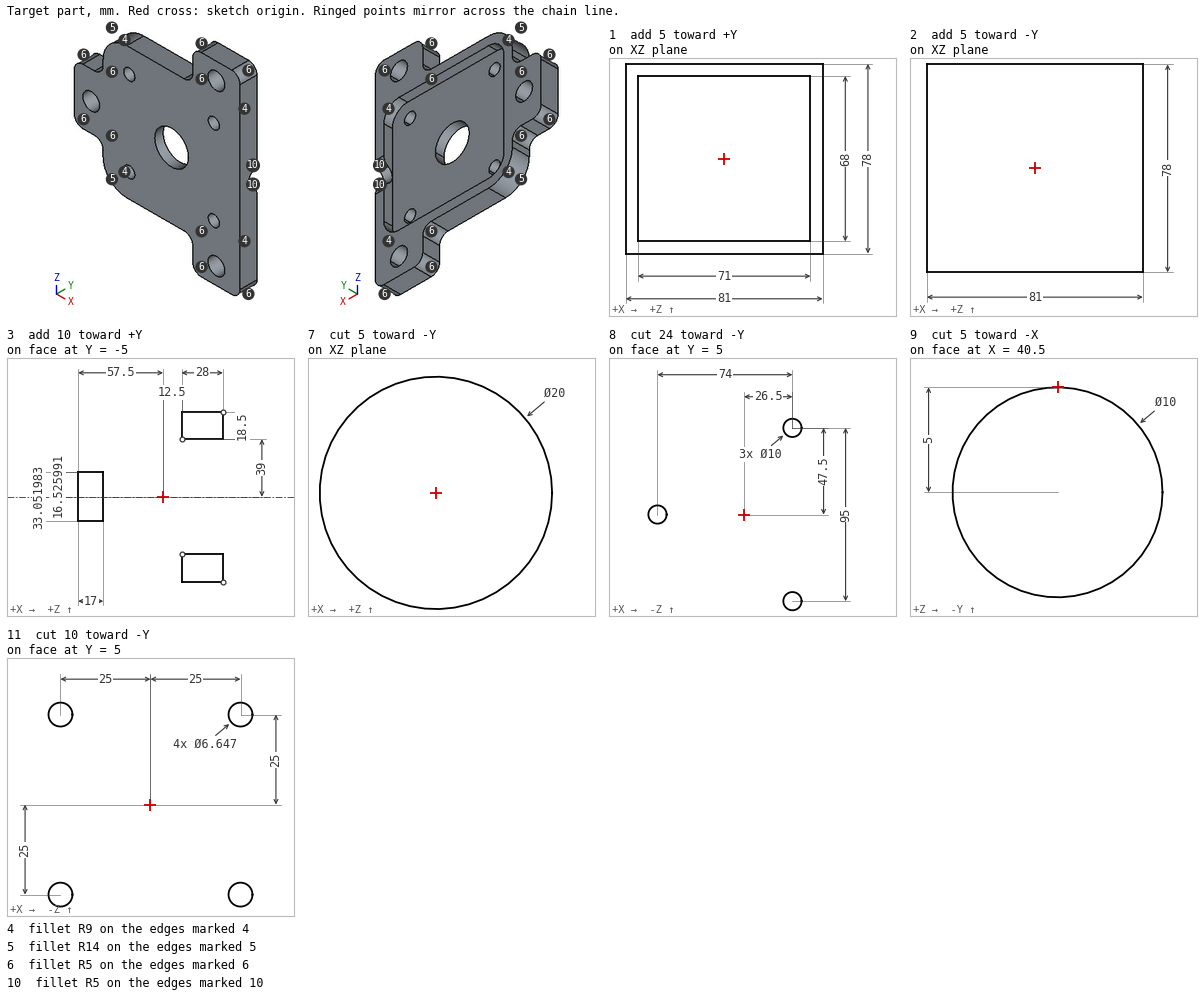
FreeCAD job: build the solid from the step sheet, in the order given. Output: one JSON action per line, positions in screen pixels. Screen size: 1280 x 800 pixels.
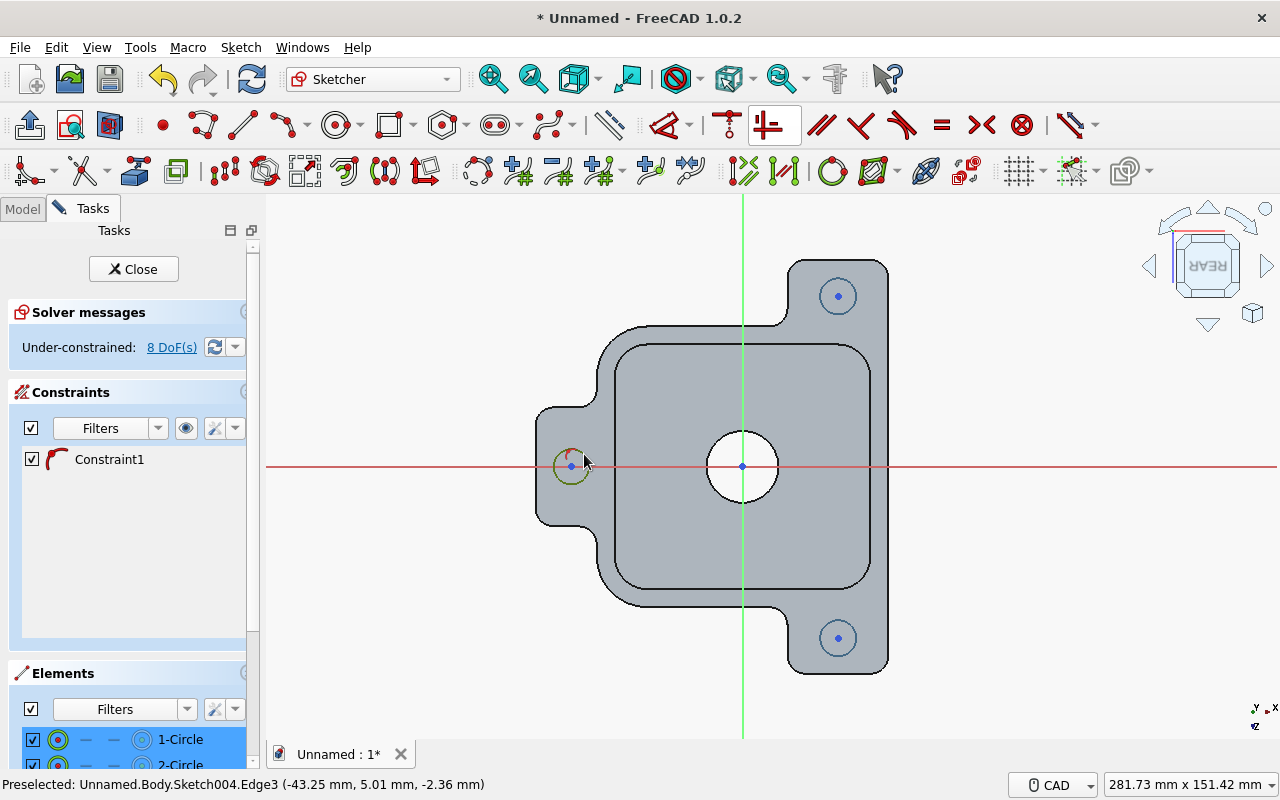
{"action": "left_click", "coordinate": [942, 126]}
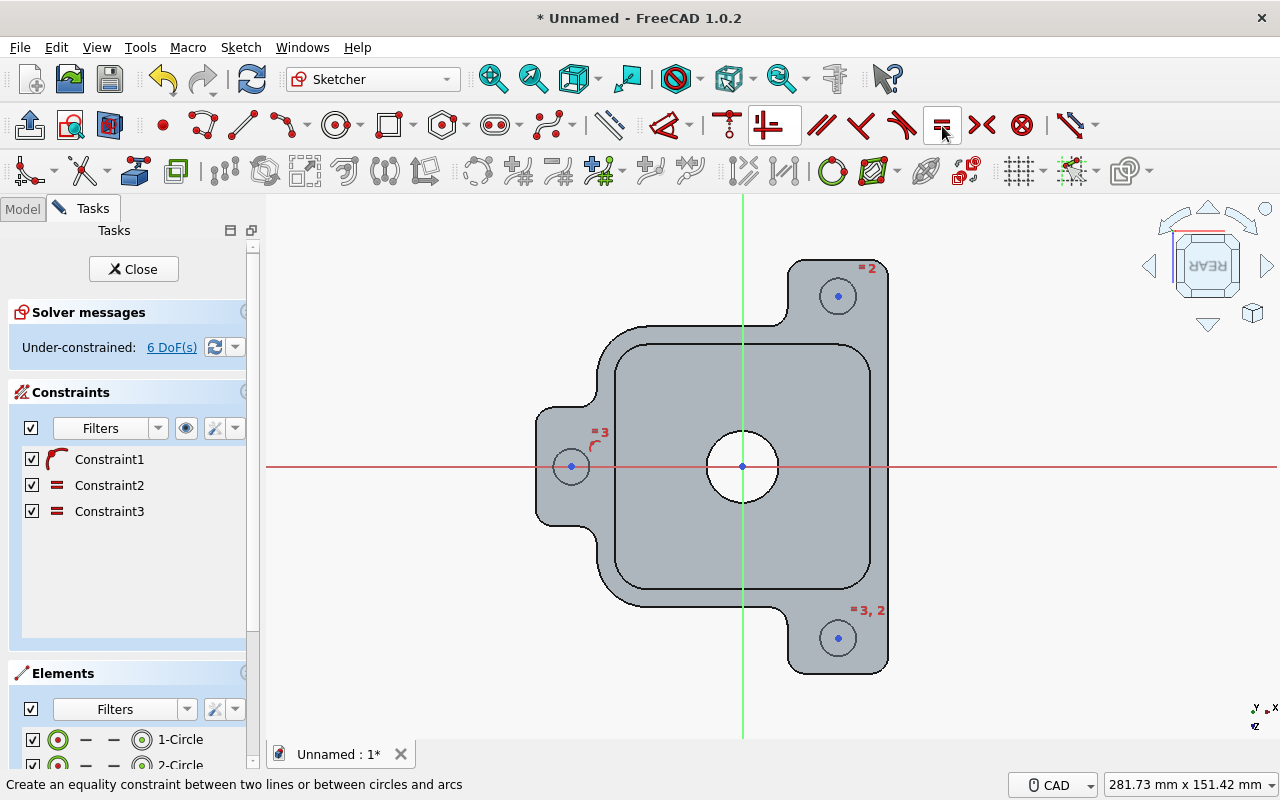
{"action": "left_click", "coordinate": [838, 296]}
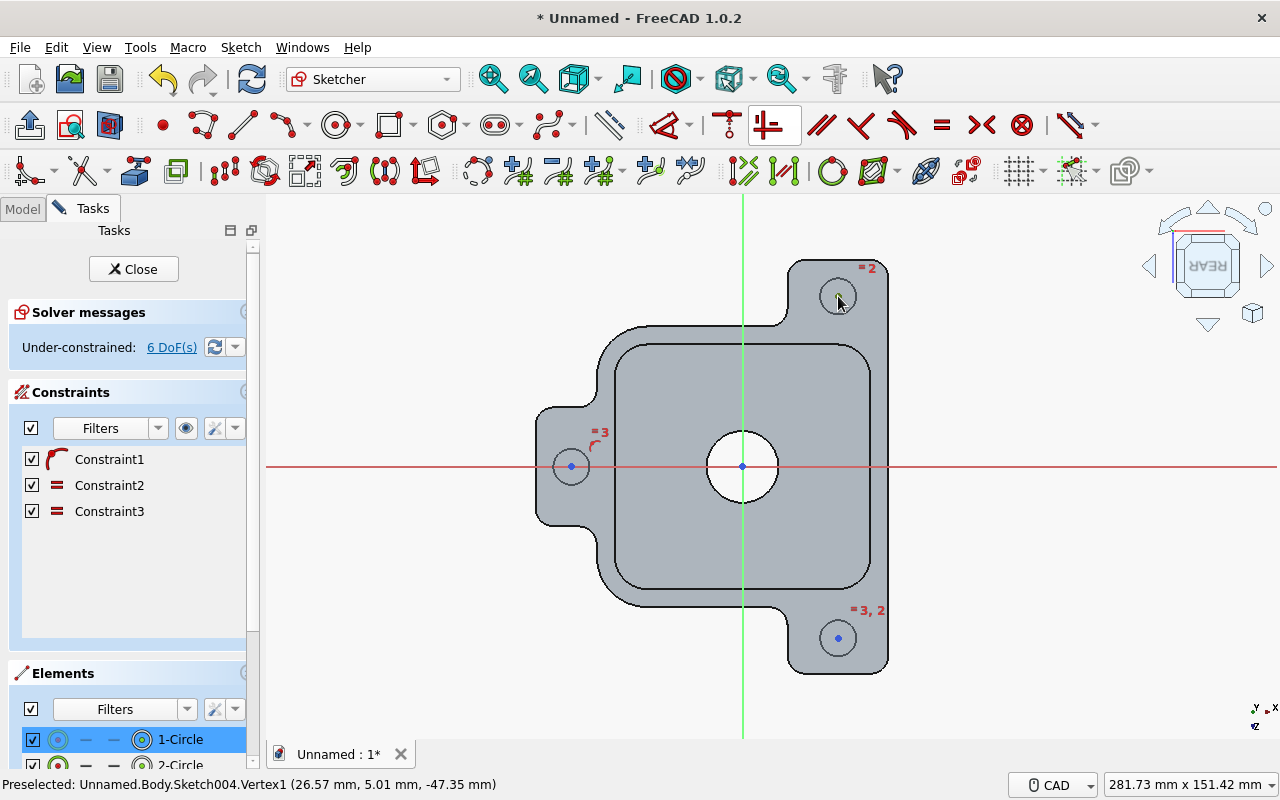
{"action": "left_click", "coordinate": [838, 638]}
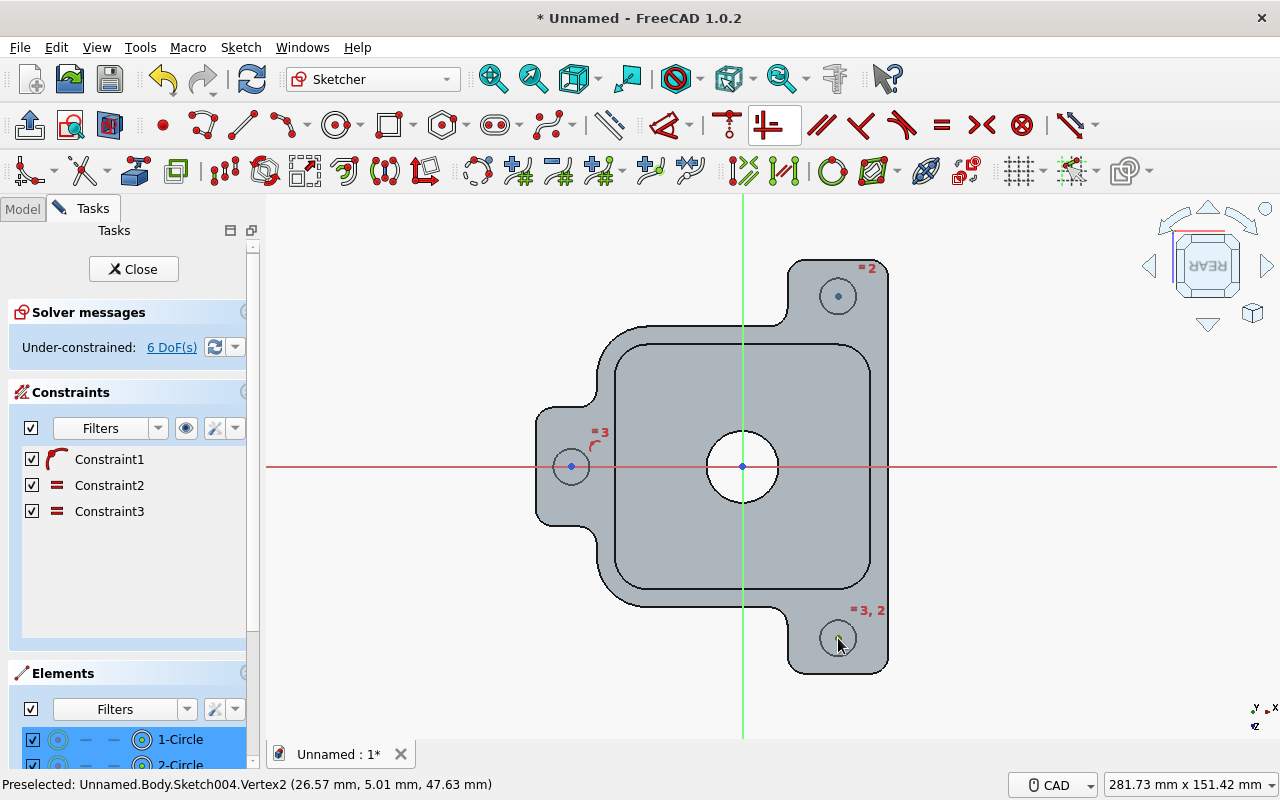
{"action": "key", "text": "v"}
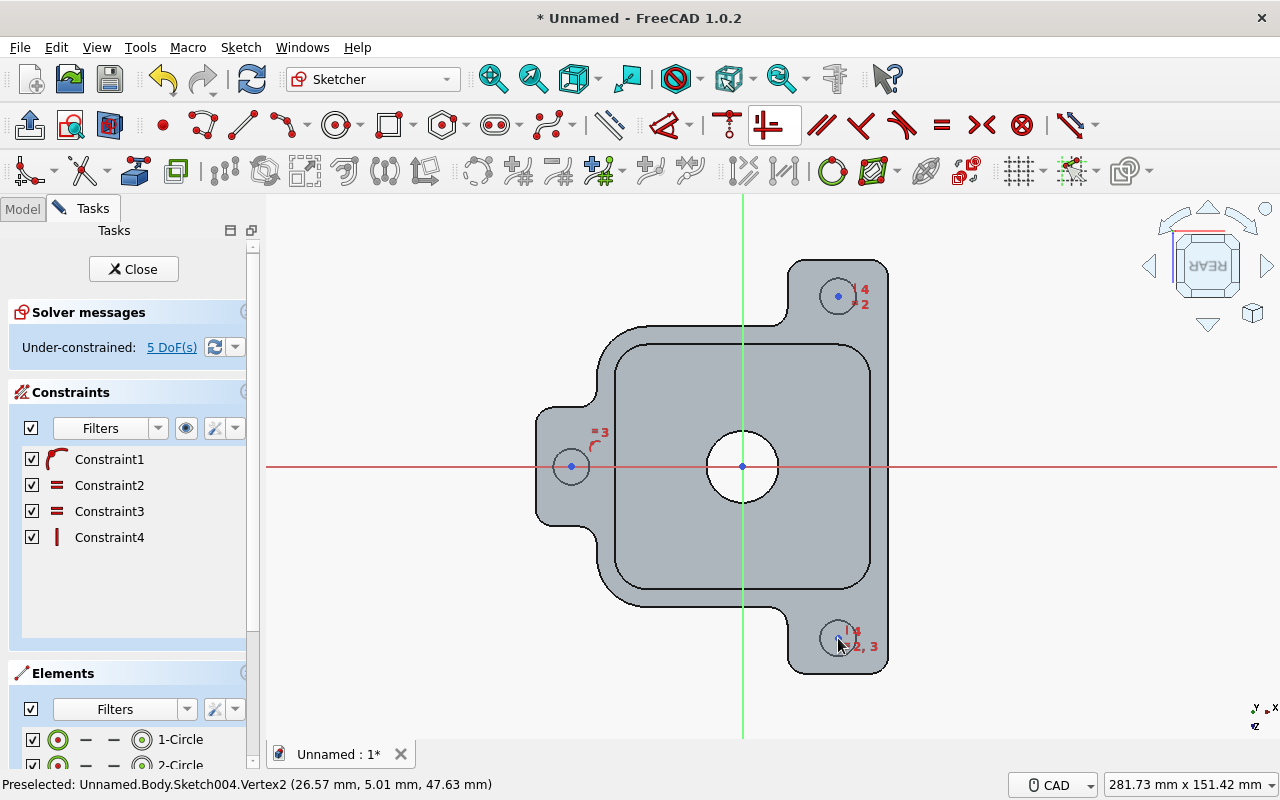
{"action": "left_click", "coordinate": [664, 126]}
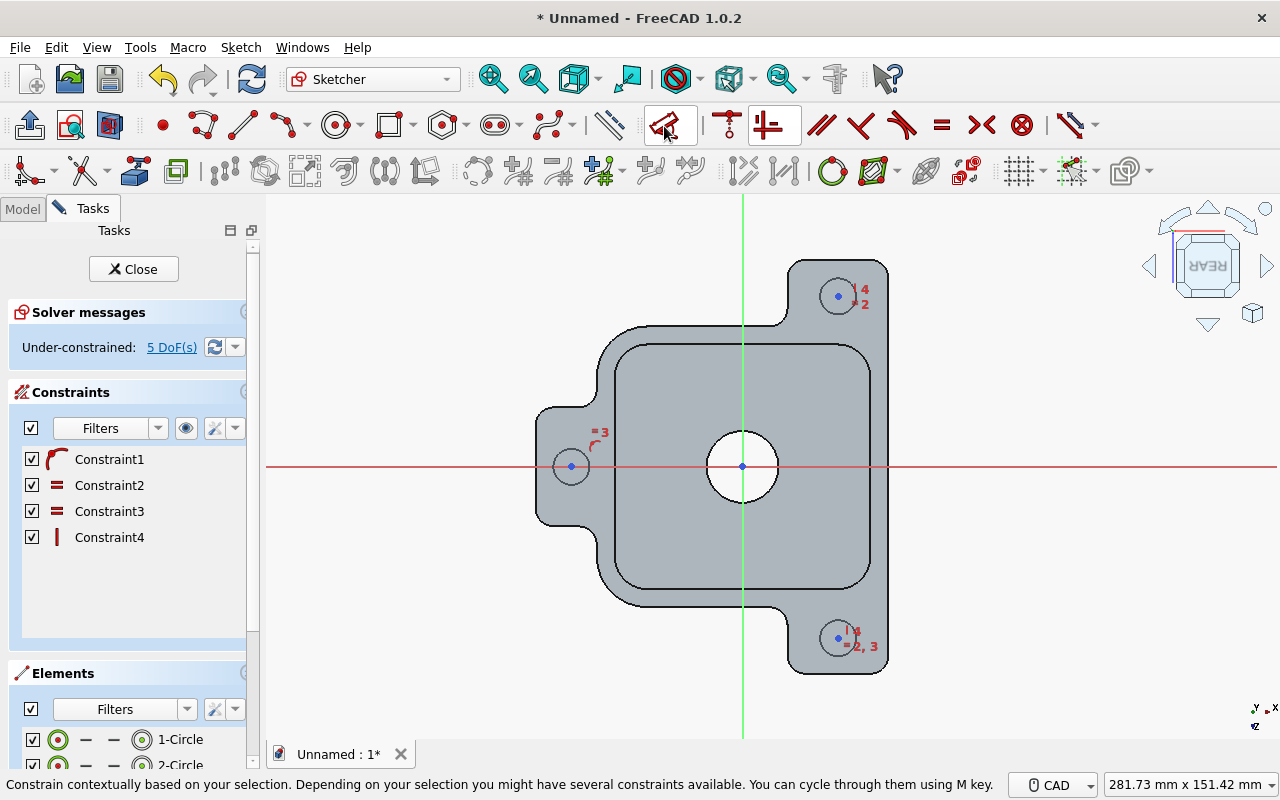
{"action": "left_click", "coordinate": [851, 284]}
{"action": "left_click", "coordinate": [874, 262]}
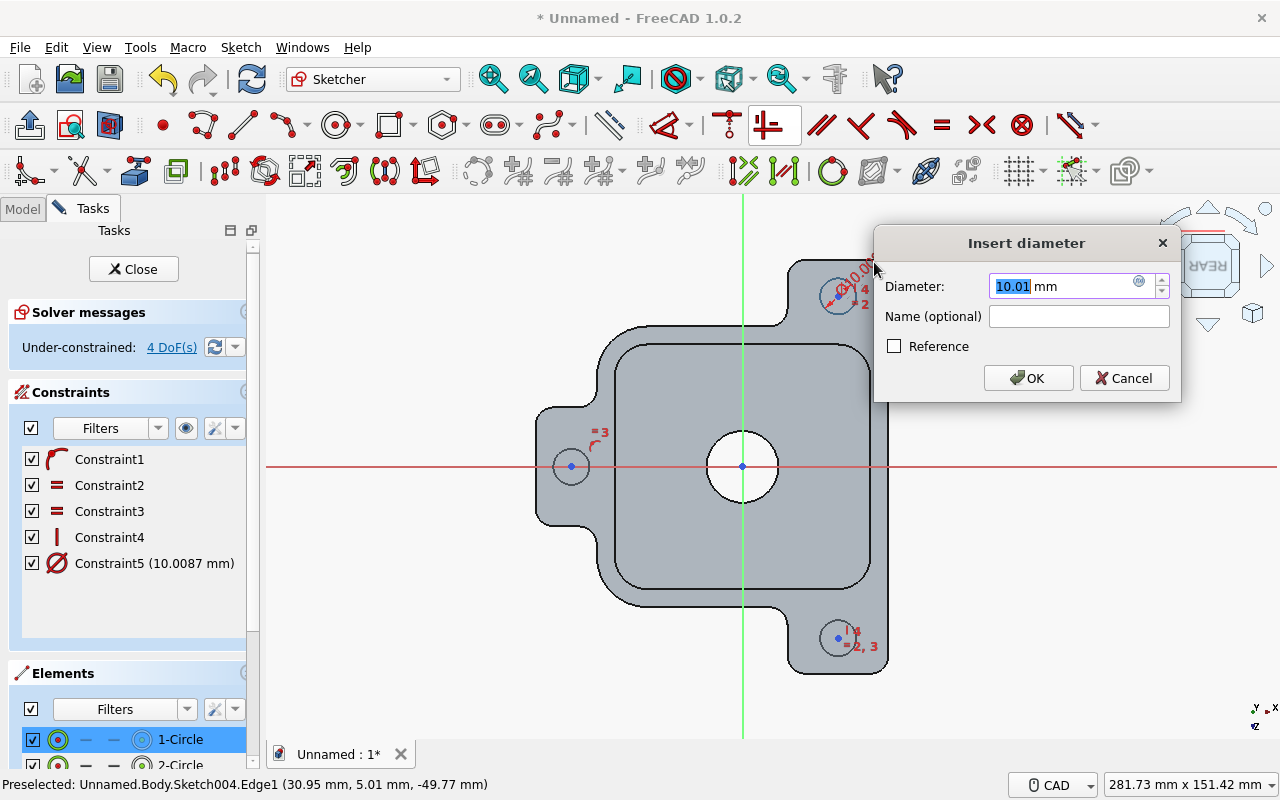
{"action": "type", "text": "10"}
{"action": "key", "text": "Return"}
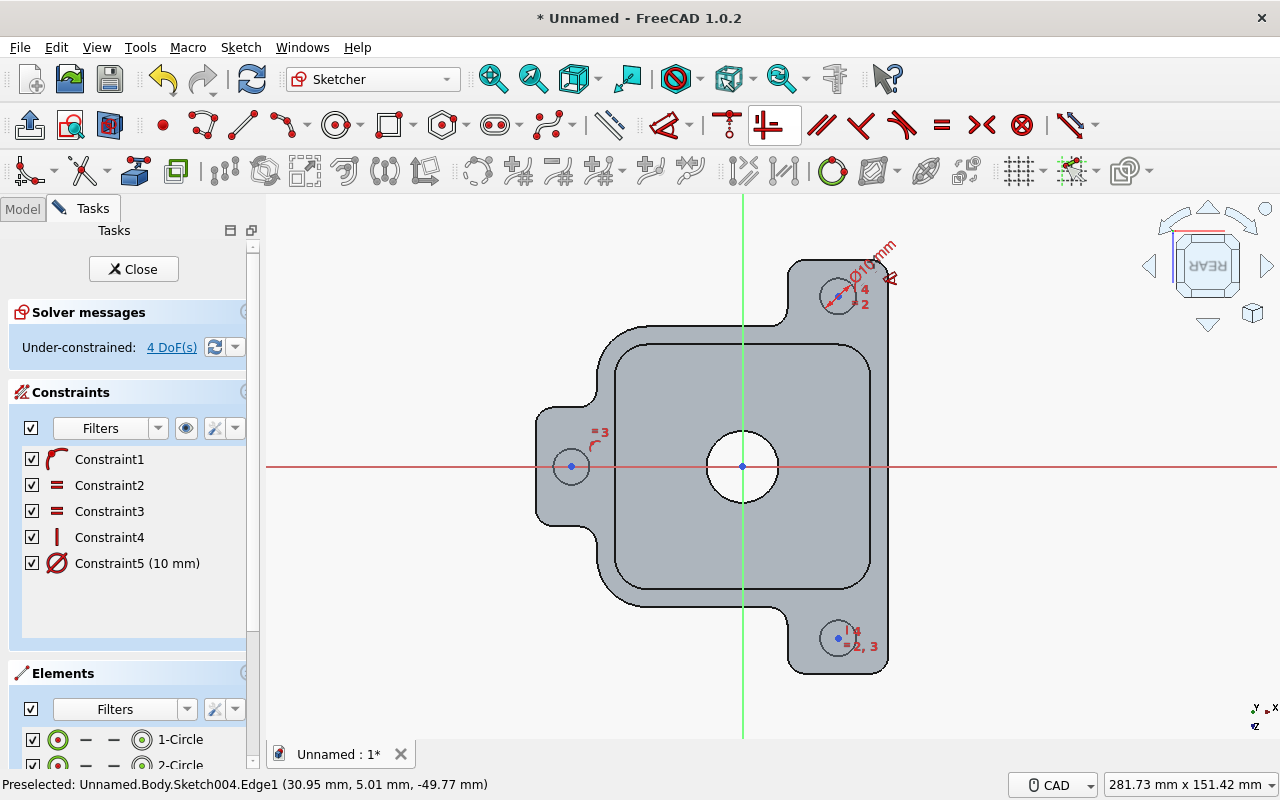
{"action": "left_click", "coordinate": [838, 296]}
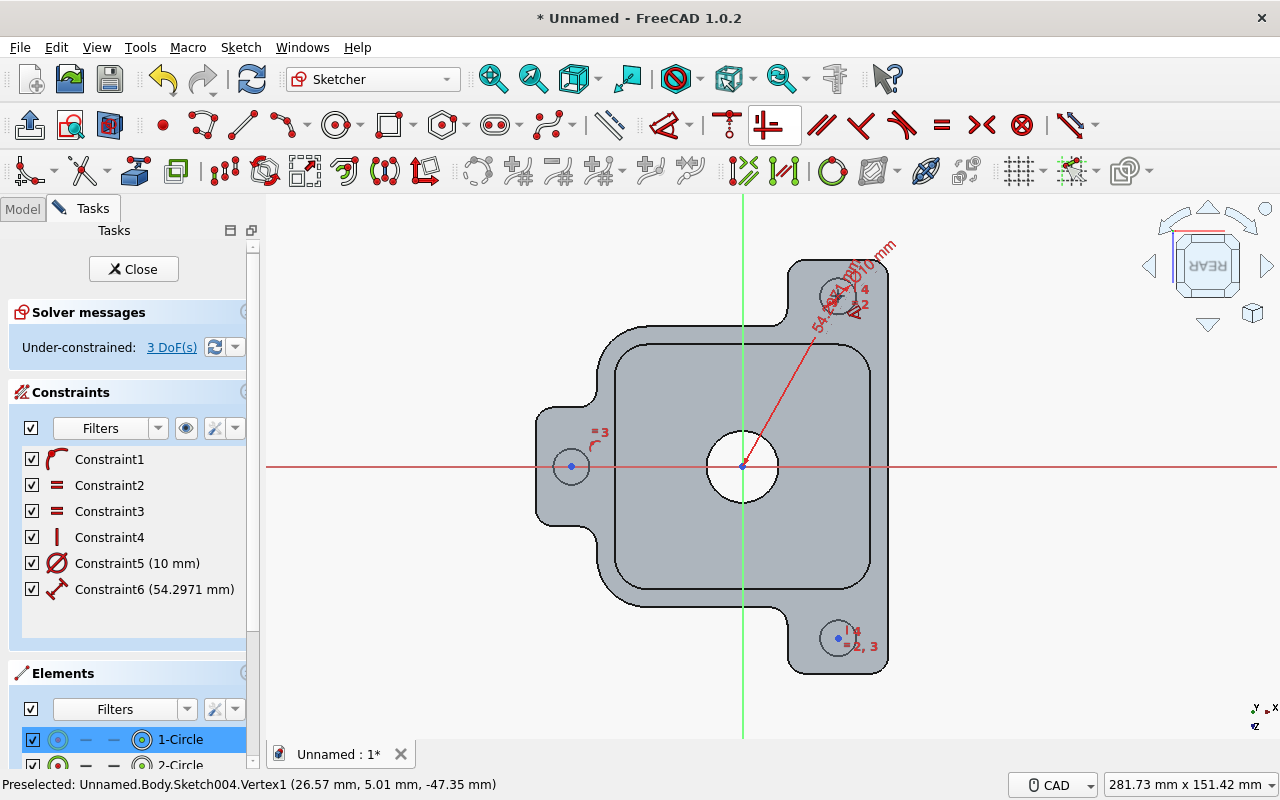
{"action": "left_click", "coordinate": [838, 638]}
{"action": "left_click", "coordinate": [872, 389]}